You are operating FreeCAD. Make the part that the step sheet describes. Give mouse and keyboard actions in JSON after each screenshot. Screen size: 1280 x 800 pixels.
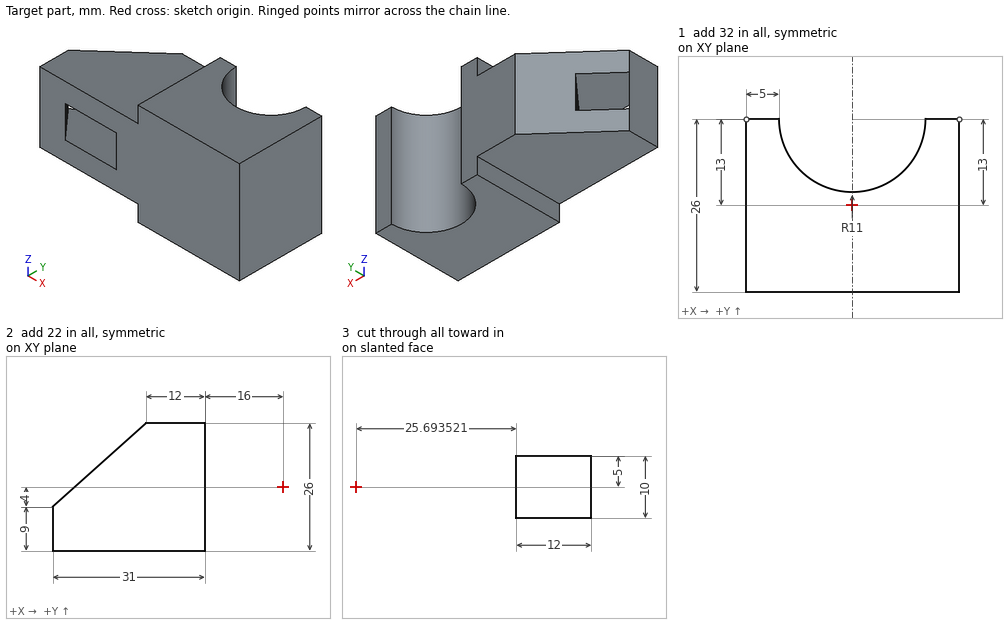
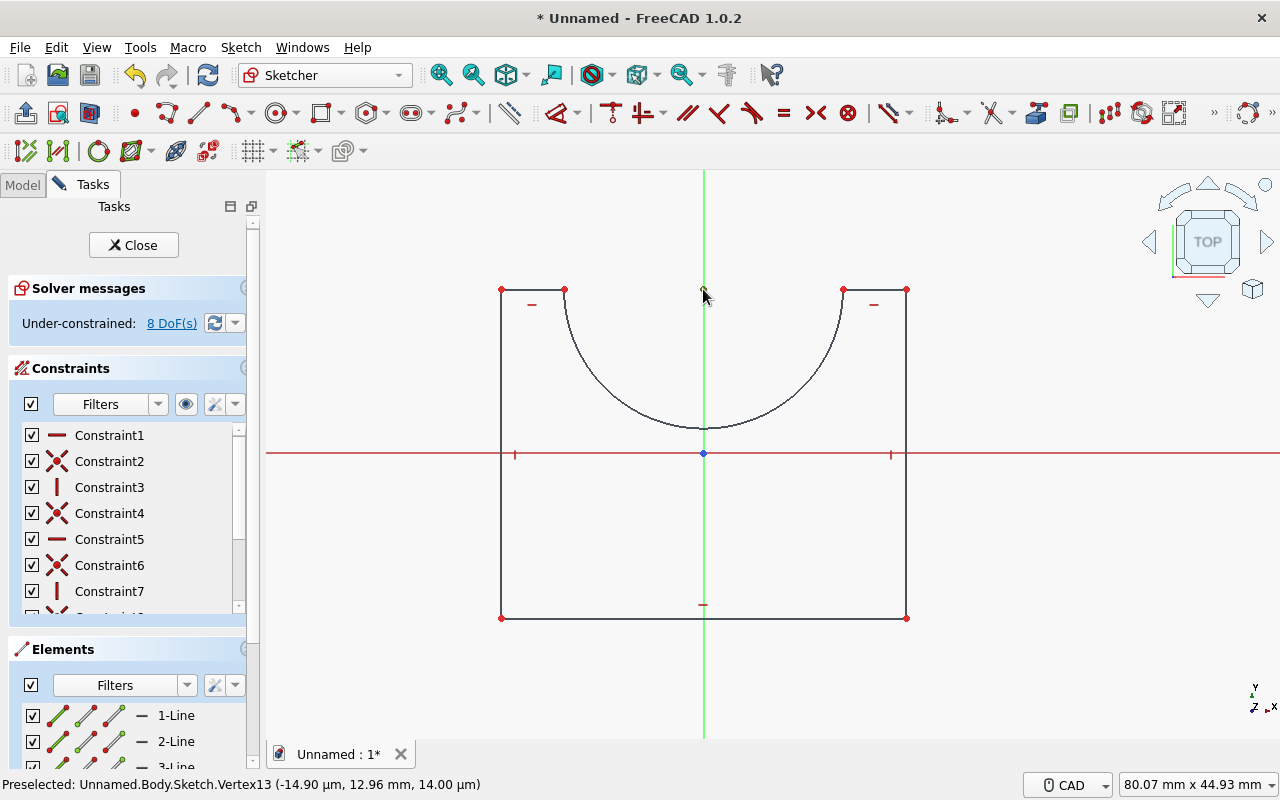
{"action": "left_click", "coordinate": [704, 674]}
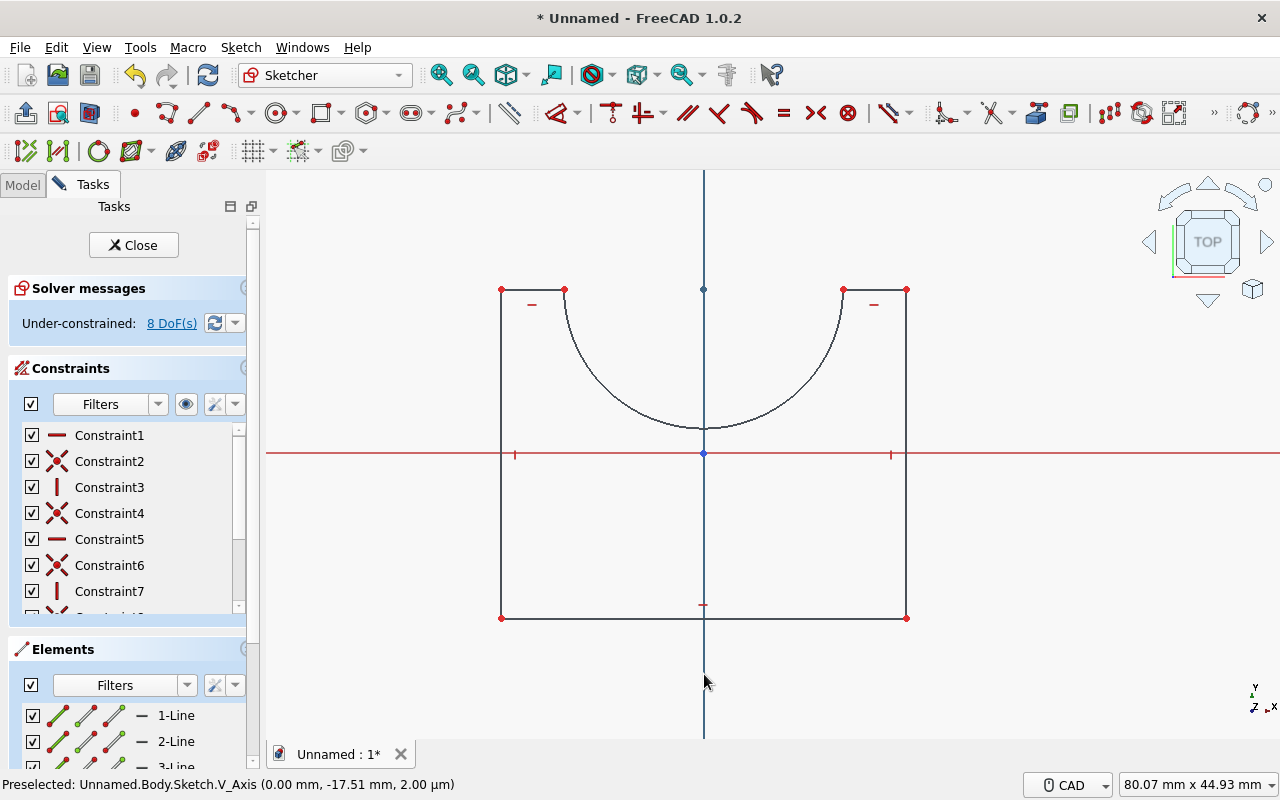
{"action": "key", "text": "c"}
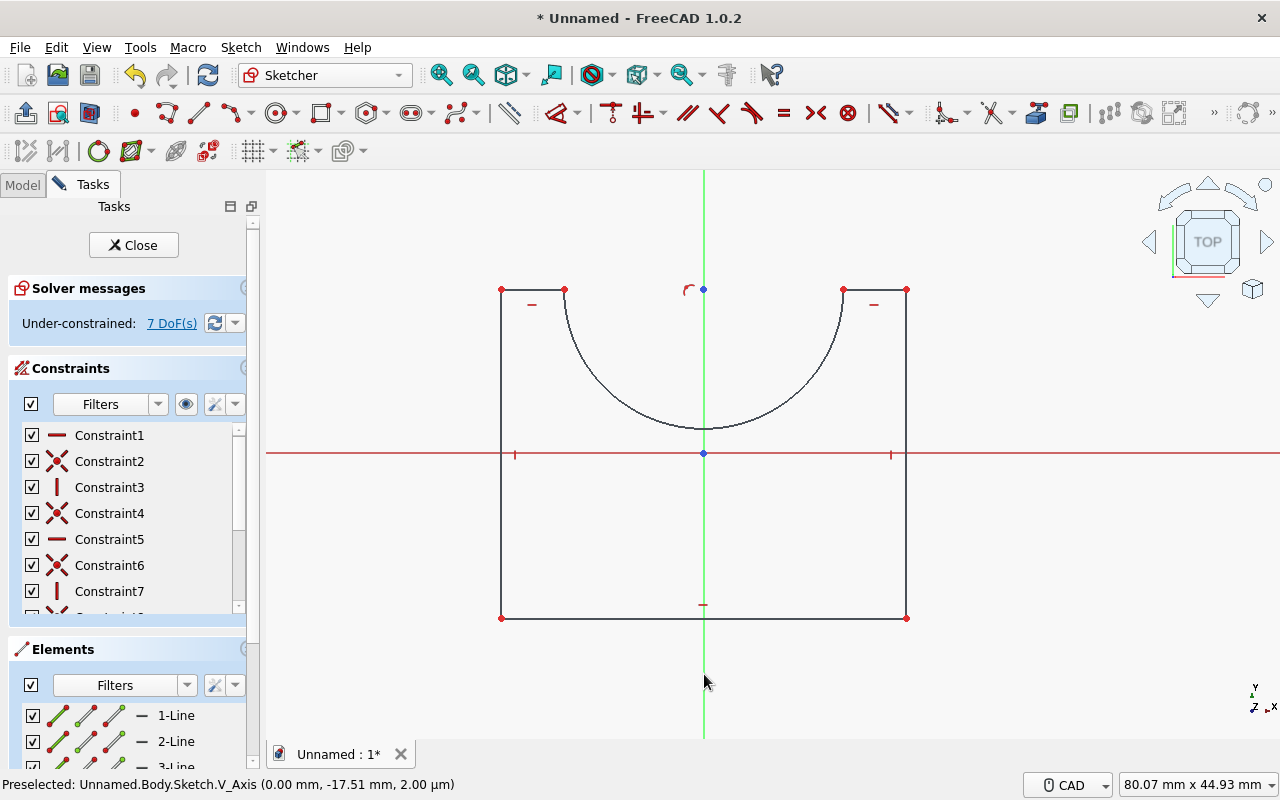
{"action": "left_click", "coordinate": [501, 290]}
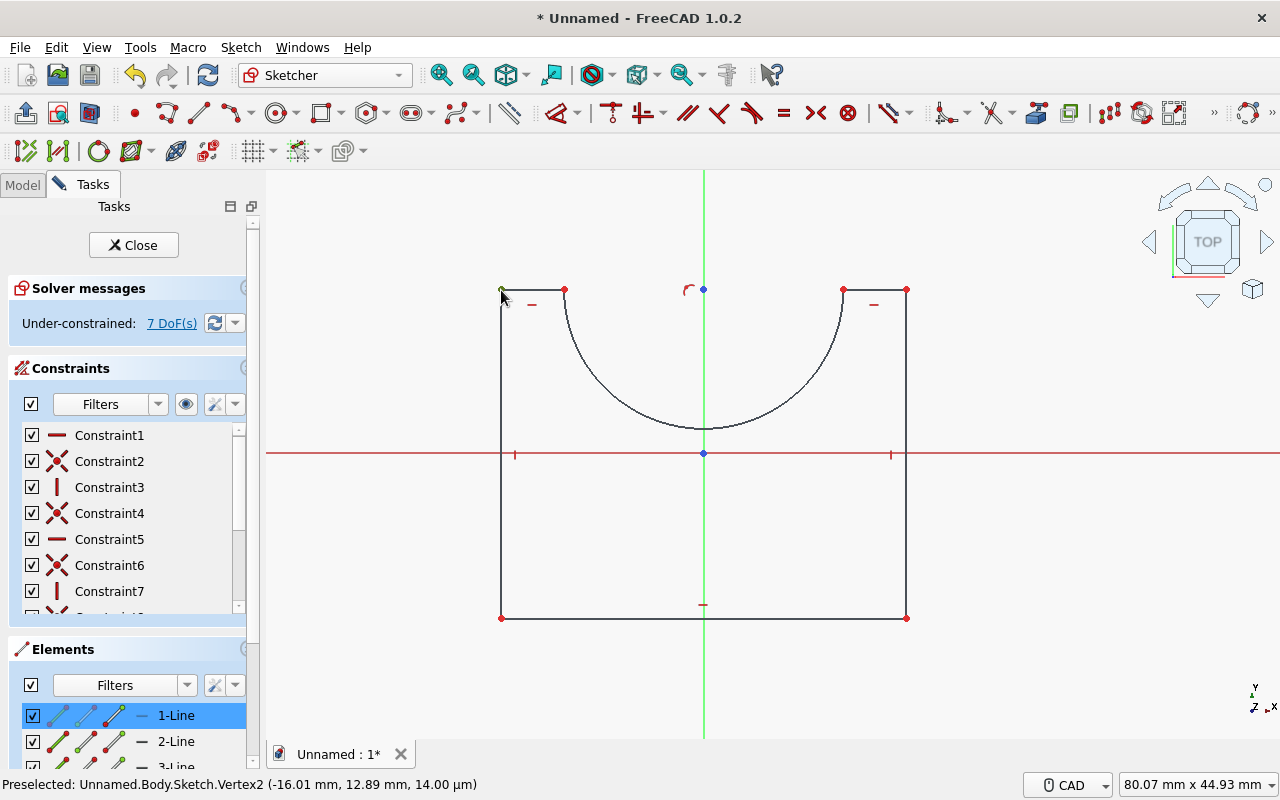
{"action": "left_click", "coordinate": [906, 290]}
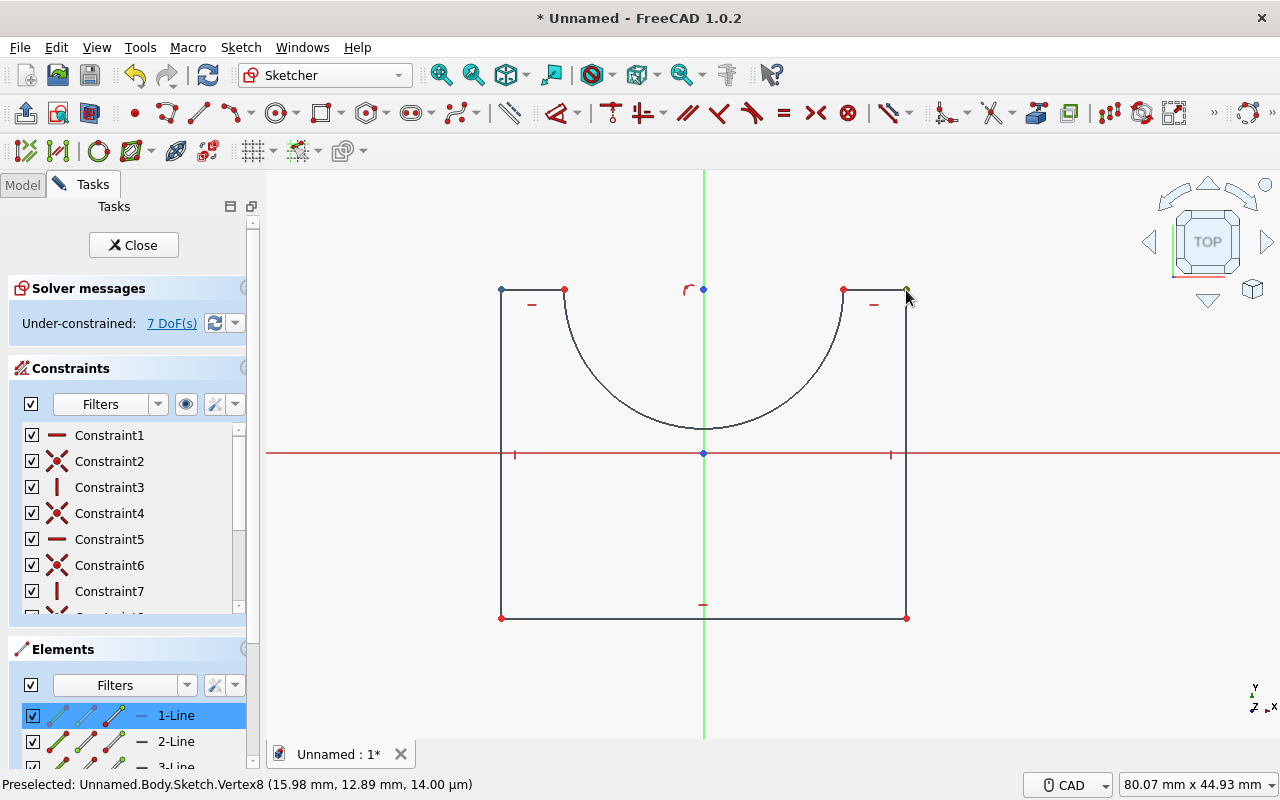
{"action": "left_click", "coordinate": [704, 674]}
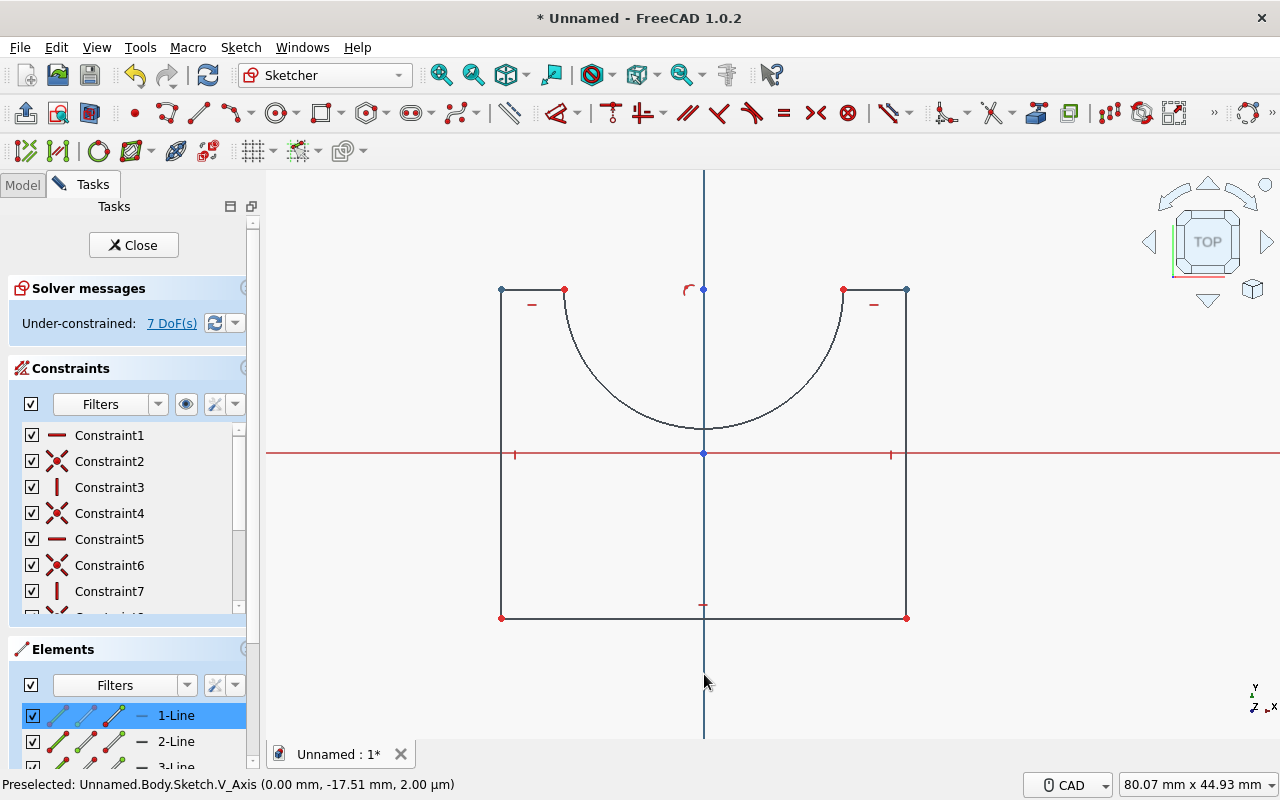
{"action": "key", "text": "s"}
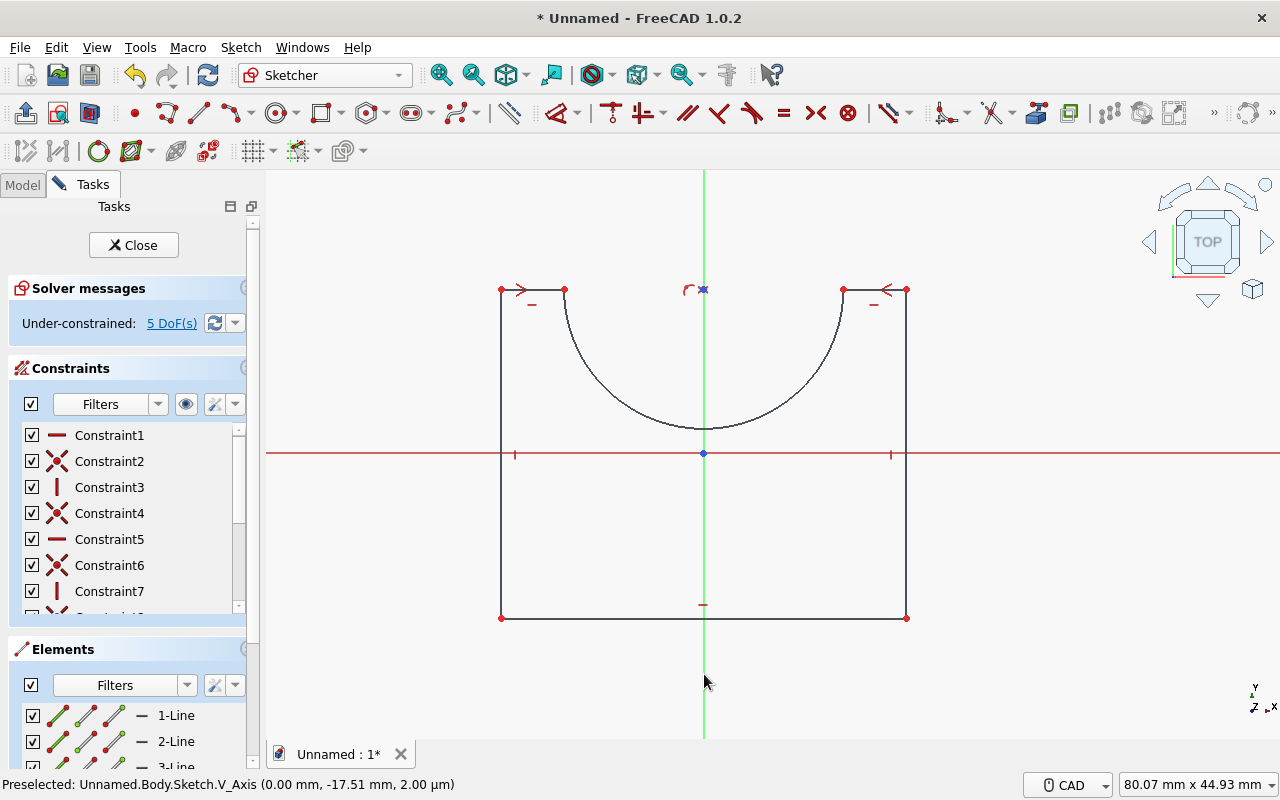
{"action": "key", "text": "d"}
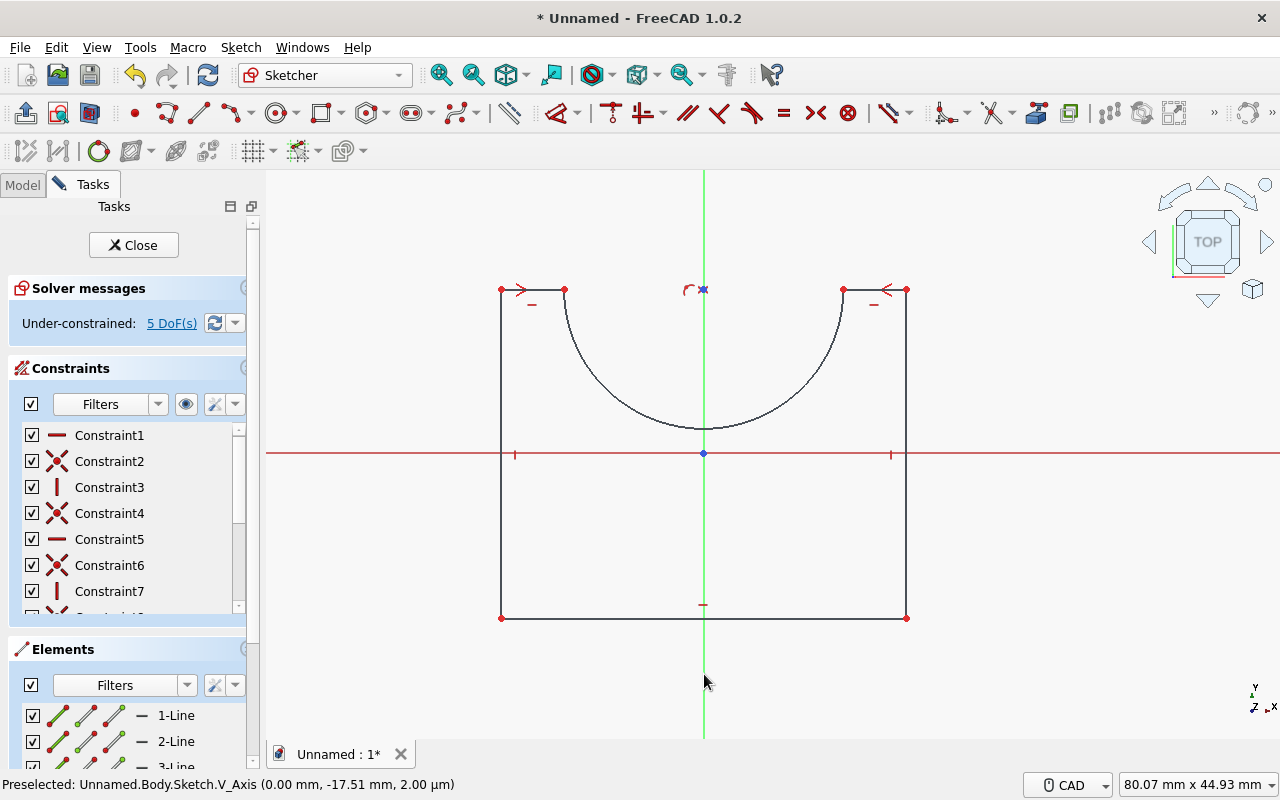
{"action": "left_click", "coordinate": [622, 402]}
{"action": "left_click", "coordinate": [603, 428]}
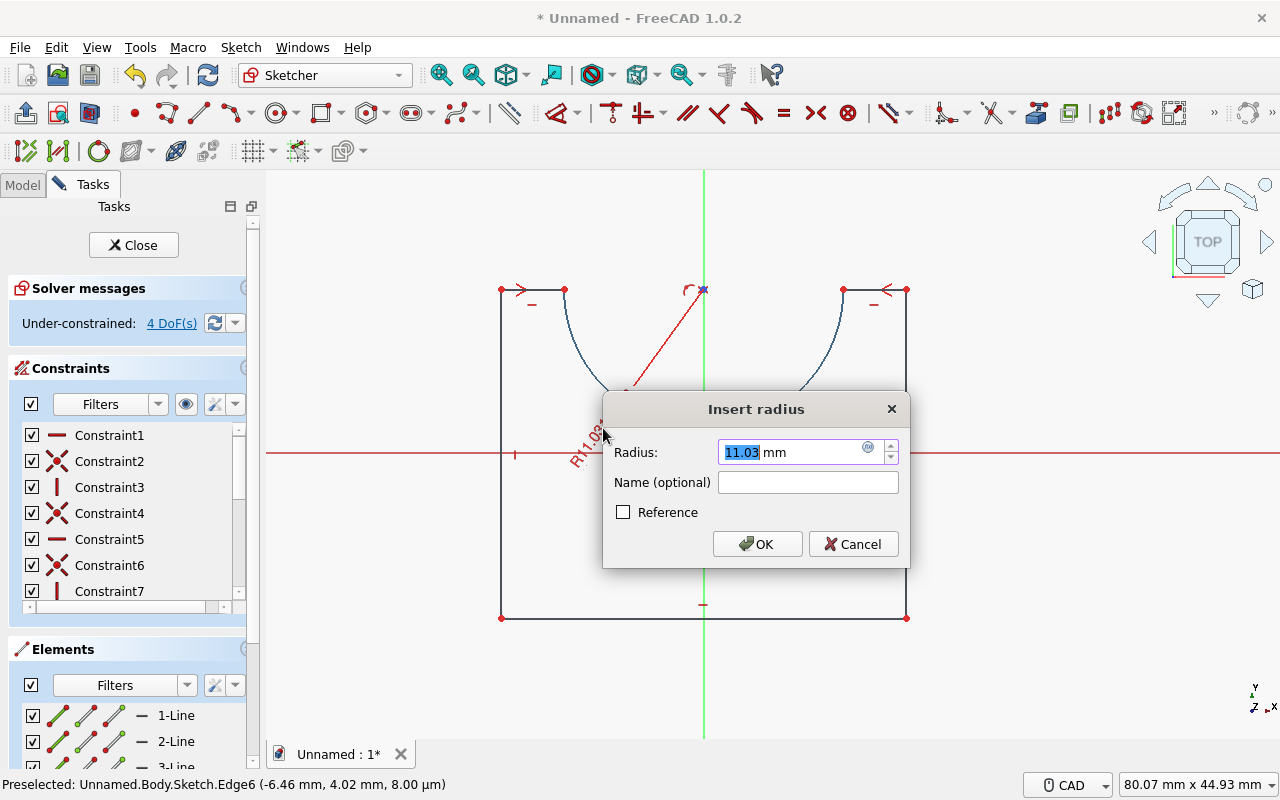
{"action": "type", "text": "11"}
{"action": "key", "text": "Return"}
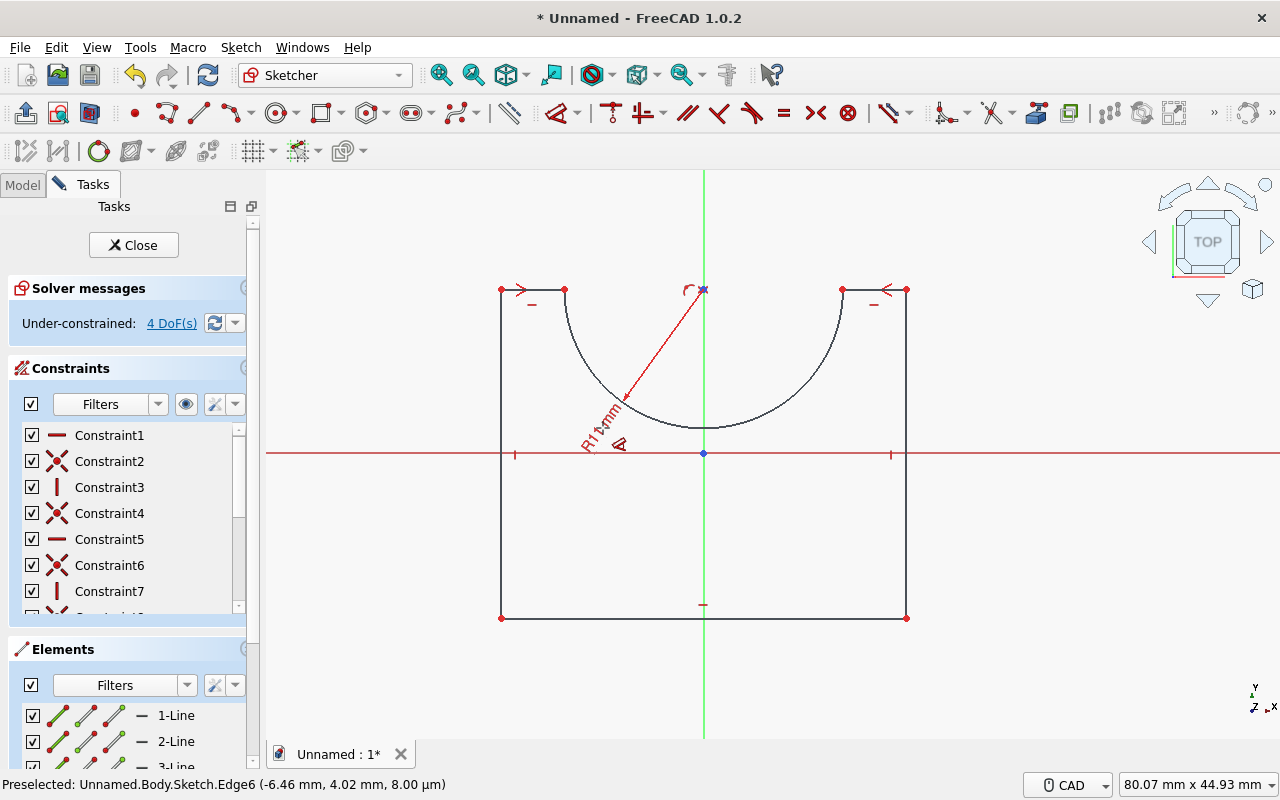
{"action": "left_click", "coordinate": [545, 290]}
{"action": "left_click", "coordinate": [533, 256]}